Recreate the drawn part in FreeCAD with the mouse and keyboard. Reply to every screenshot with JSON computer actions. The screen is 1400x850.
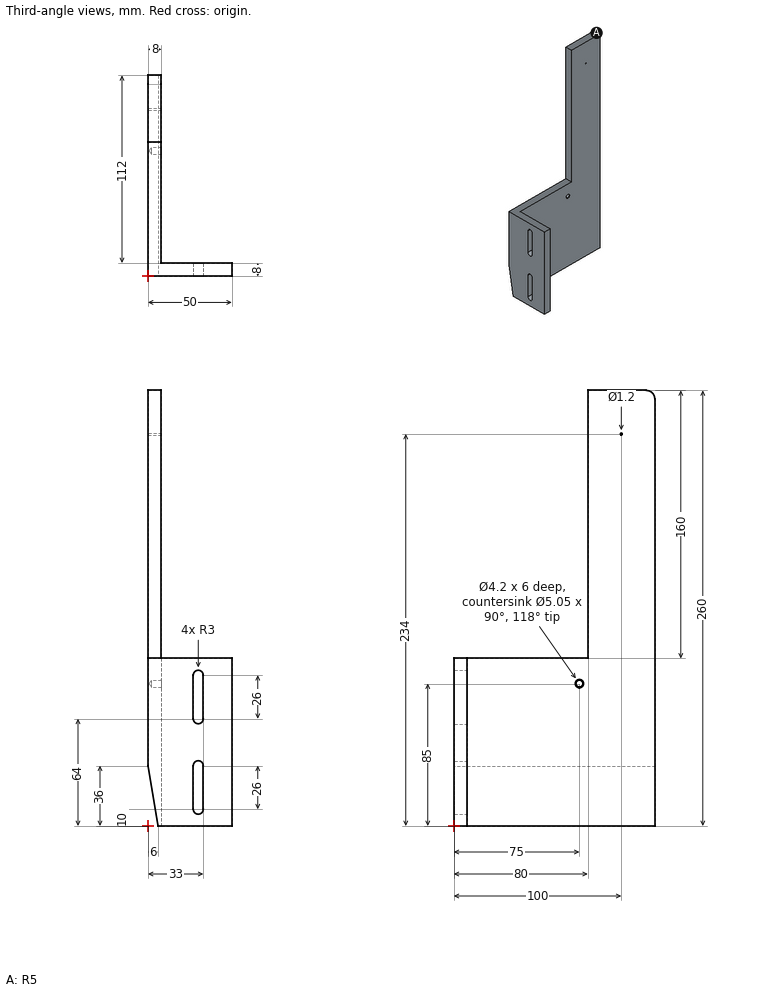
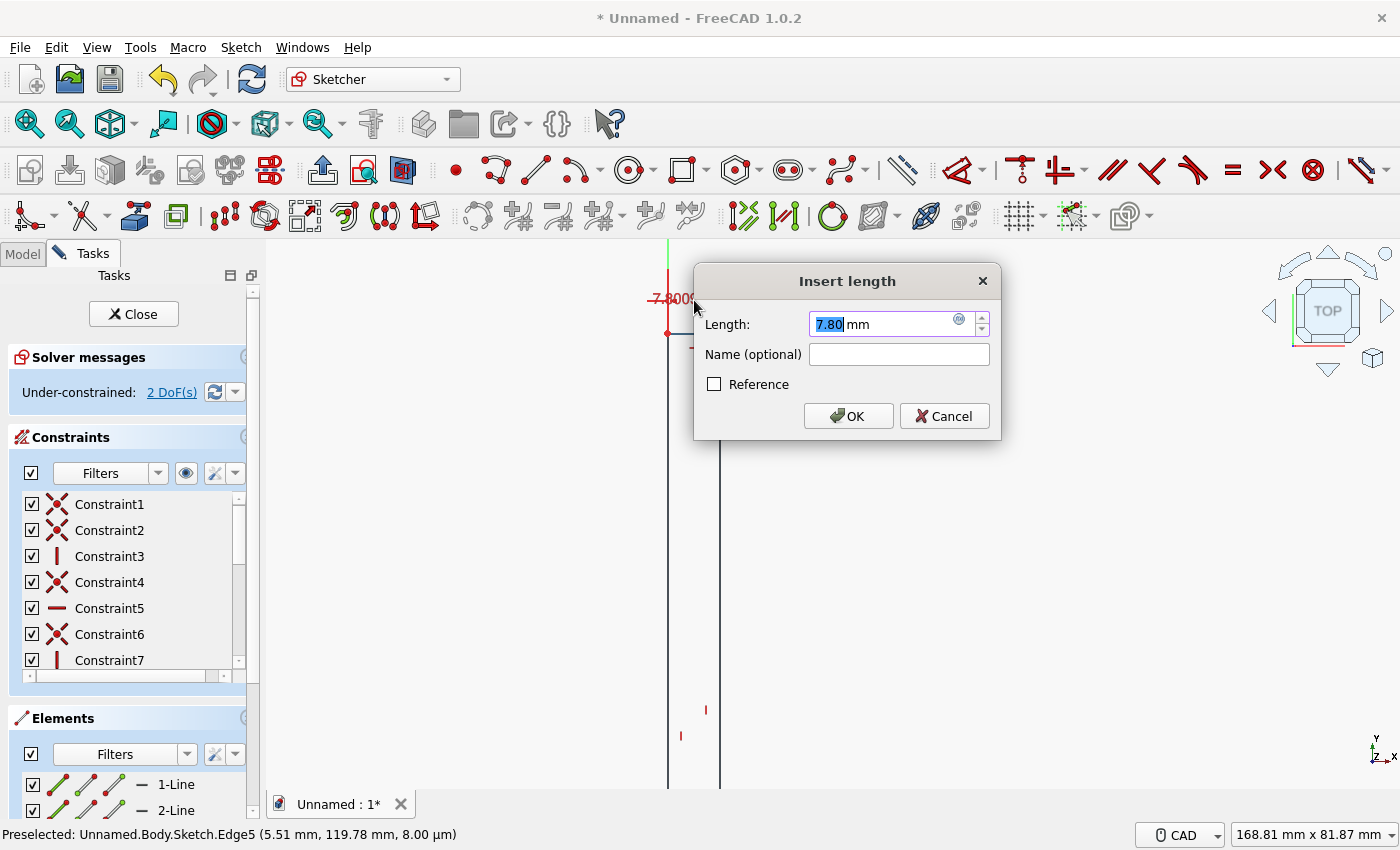
{"action": "type", "text": "8"}
{"action": "key", "text": "Return"}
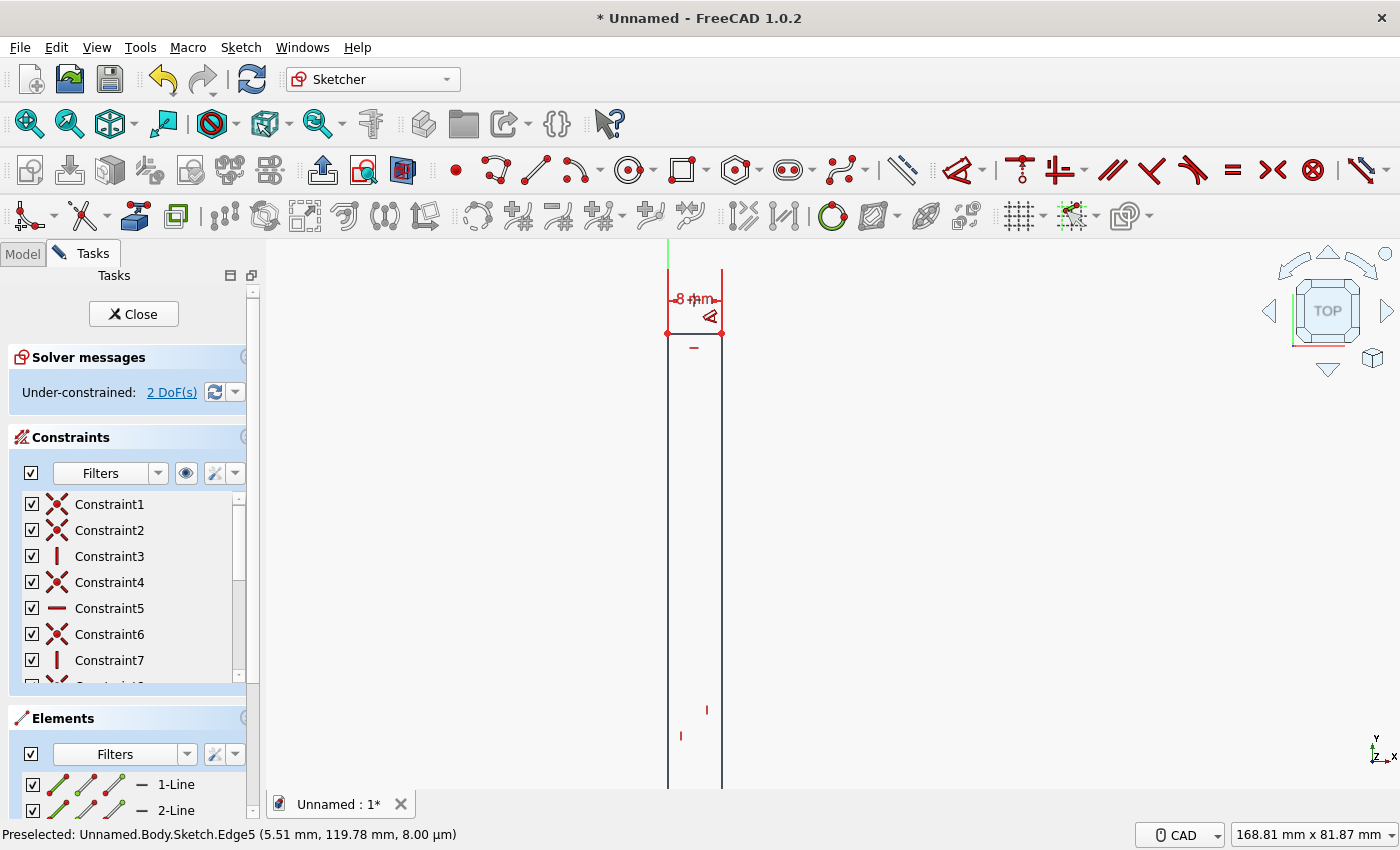
{"action": "scroll", "coordinate": [706, 333], "scroll_direction": "down", "scroll_amount": 4}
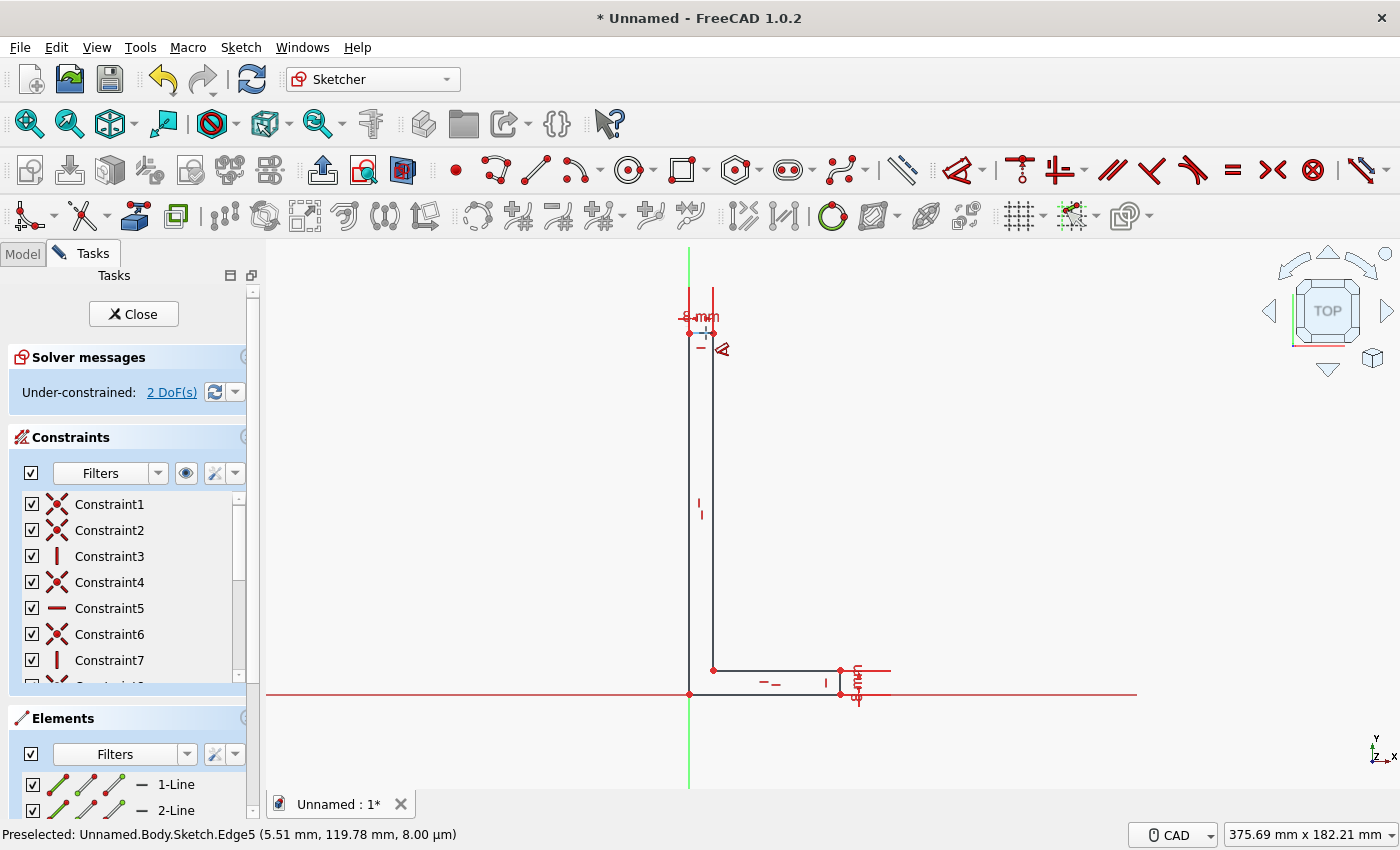
{"action": "left_click", "coordinate": [735, 695]}
{"action": "left_click", "coordinate": [765, 729]}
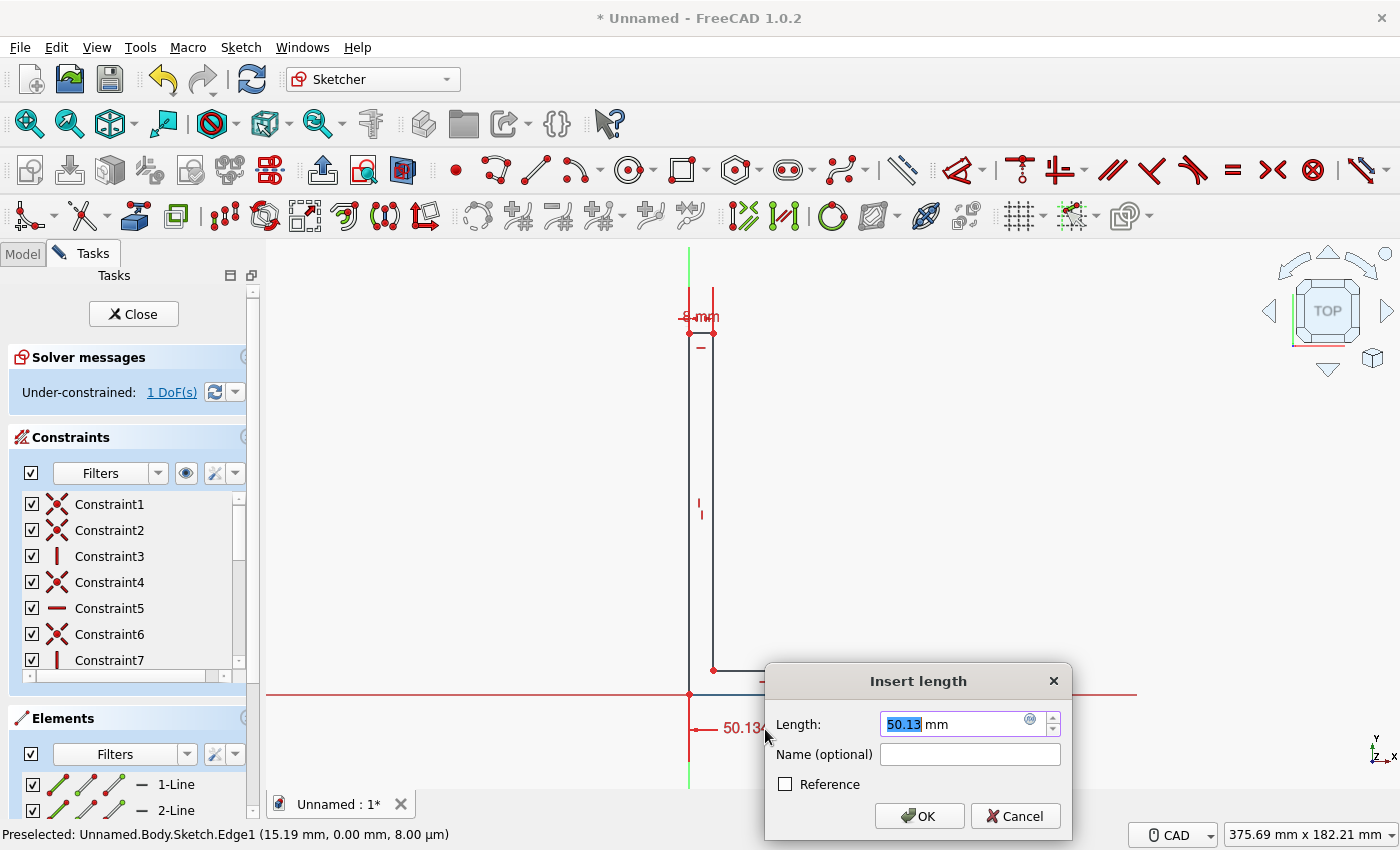
{"action": "type", "text": "50"}
{"action": "key", "text": "Return"}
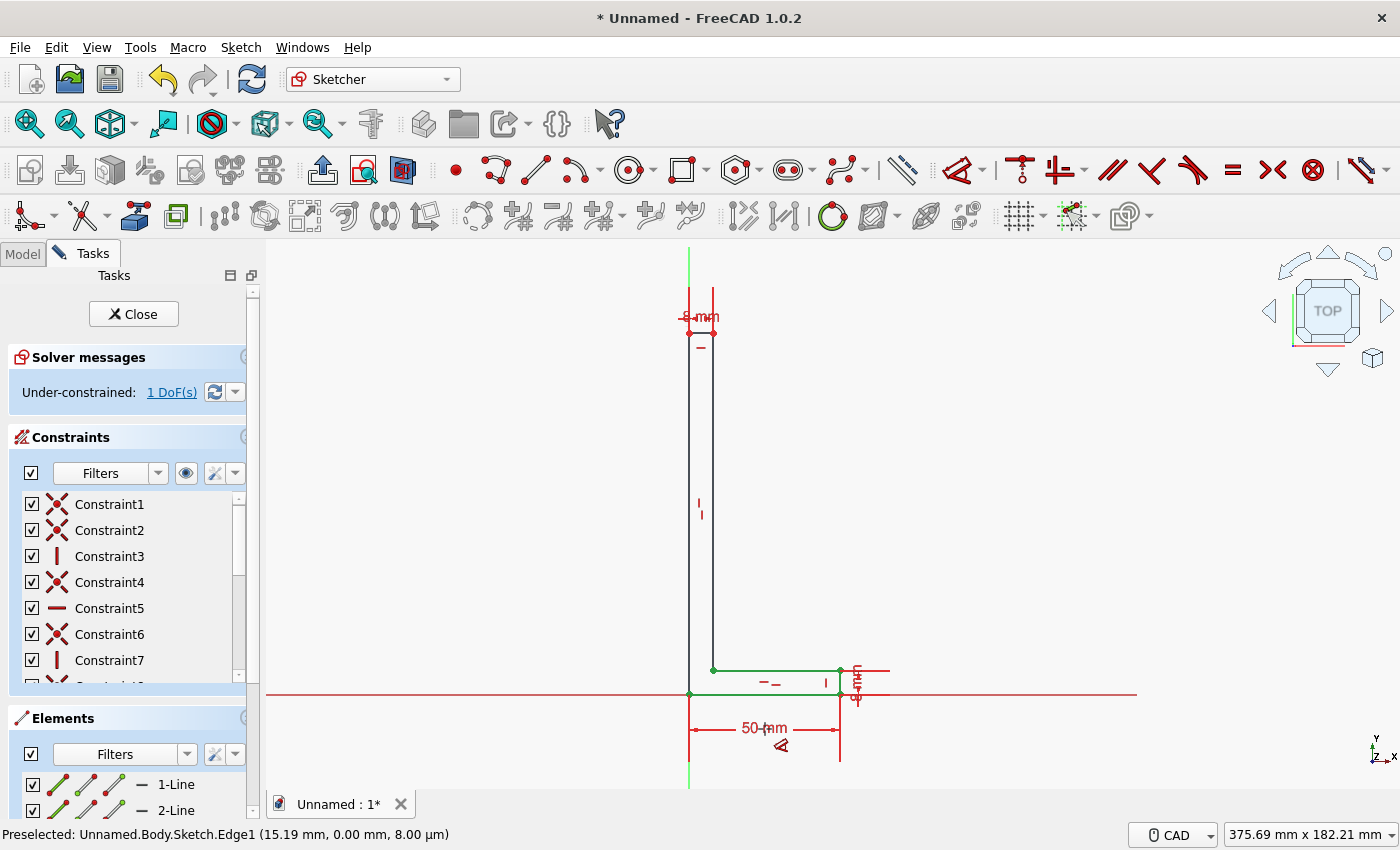
{"action": "left_click", "coordinate": [713, 570]}
{"action": "left_click", "coordinate": [747, 502]}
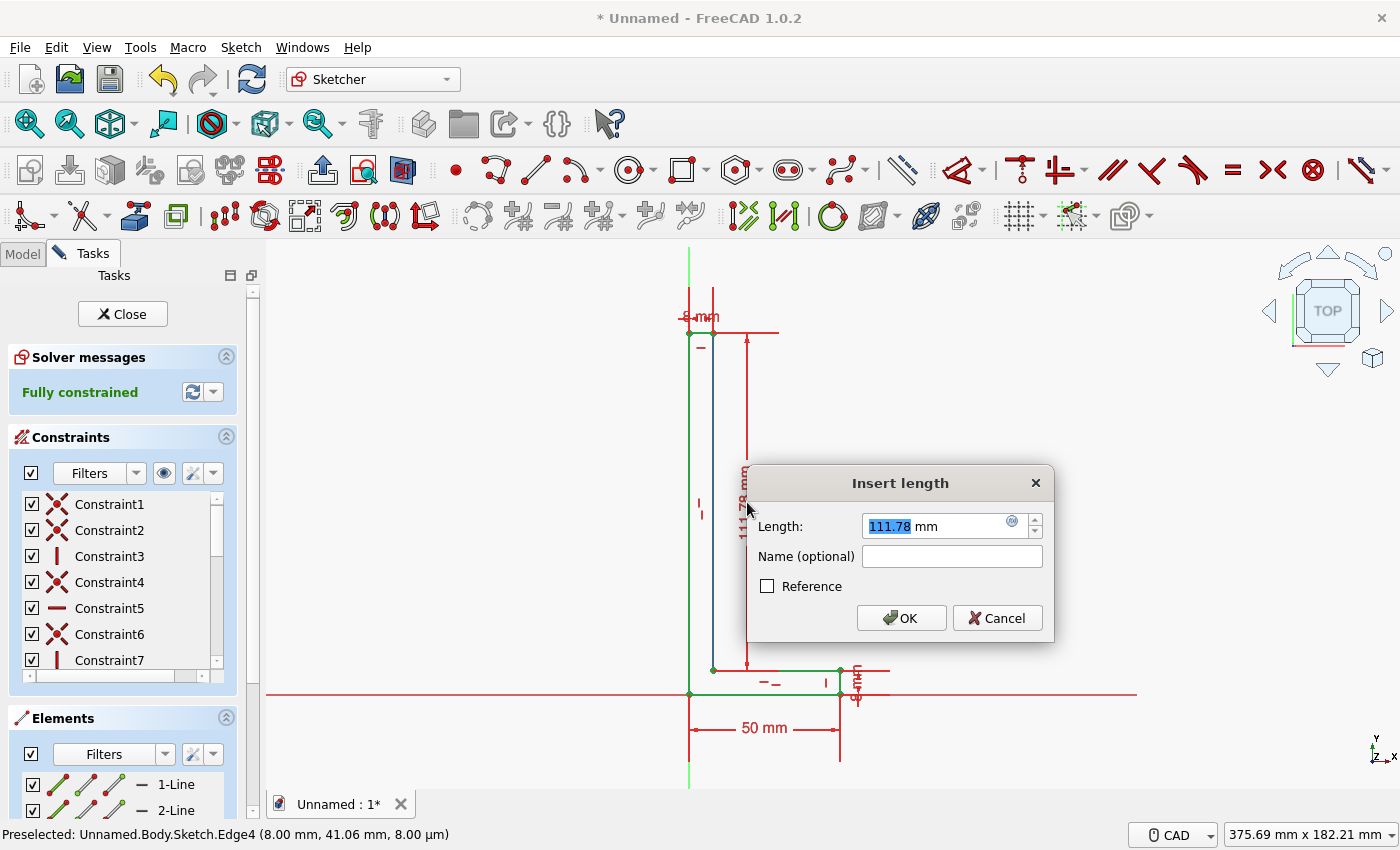
{"action": "type", "text": "112"}
{"action": "key", "text": "Return"}
{"action": "key", "text": "Escape"}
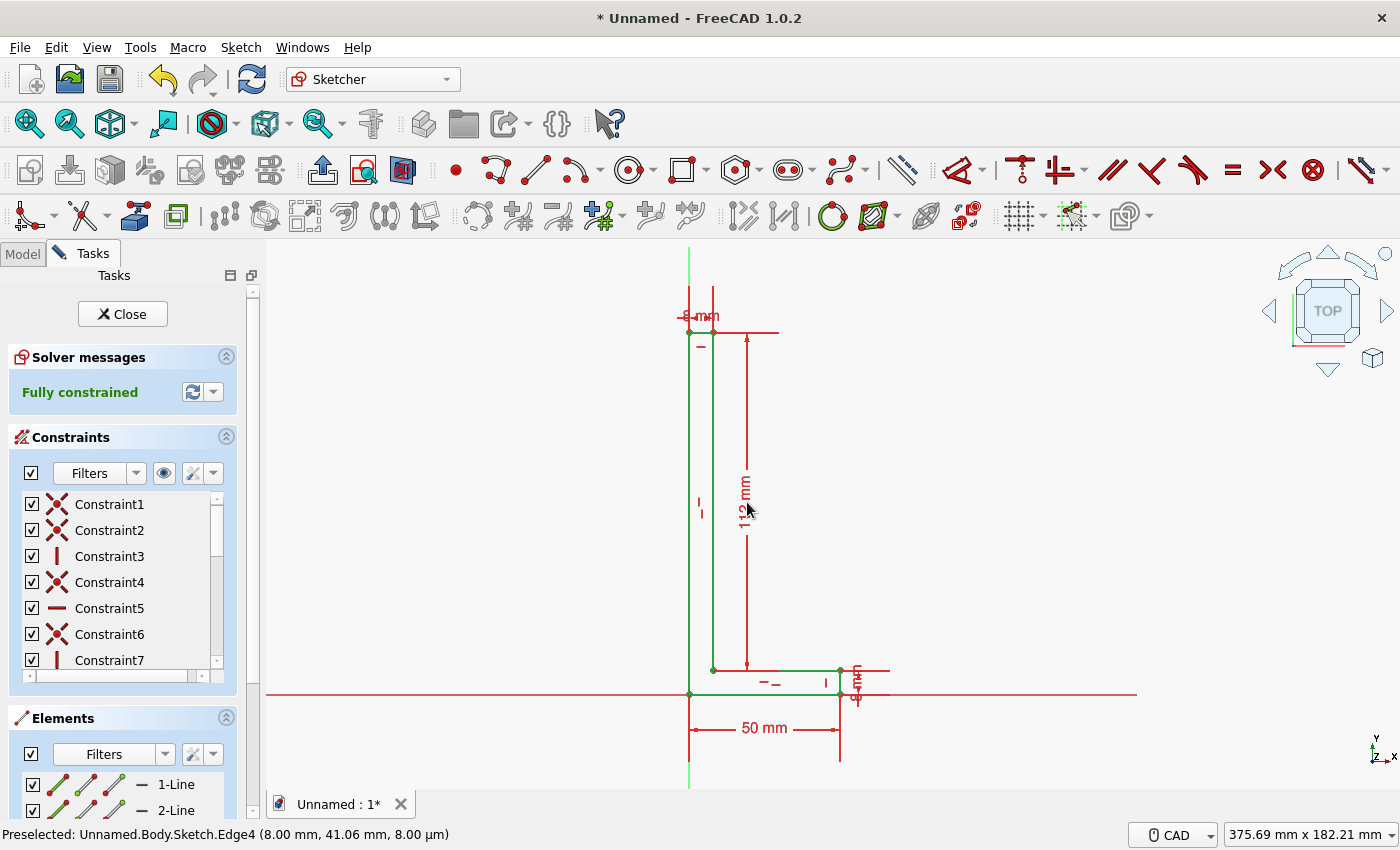
{"action": "left_click", "coordinate": [123, 314]}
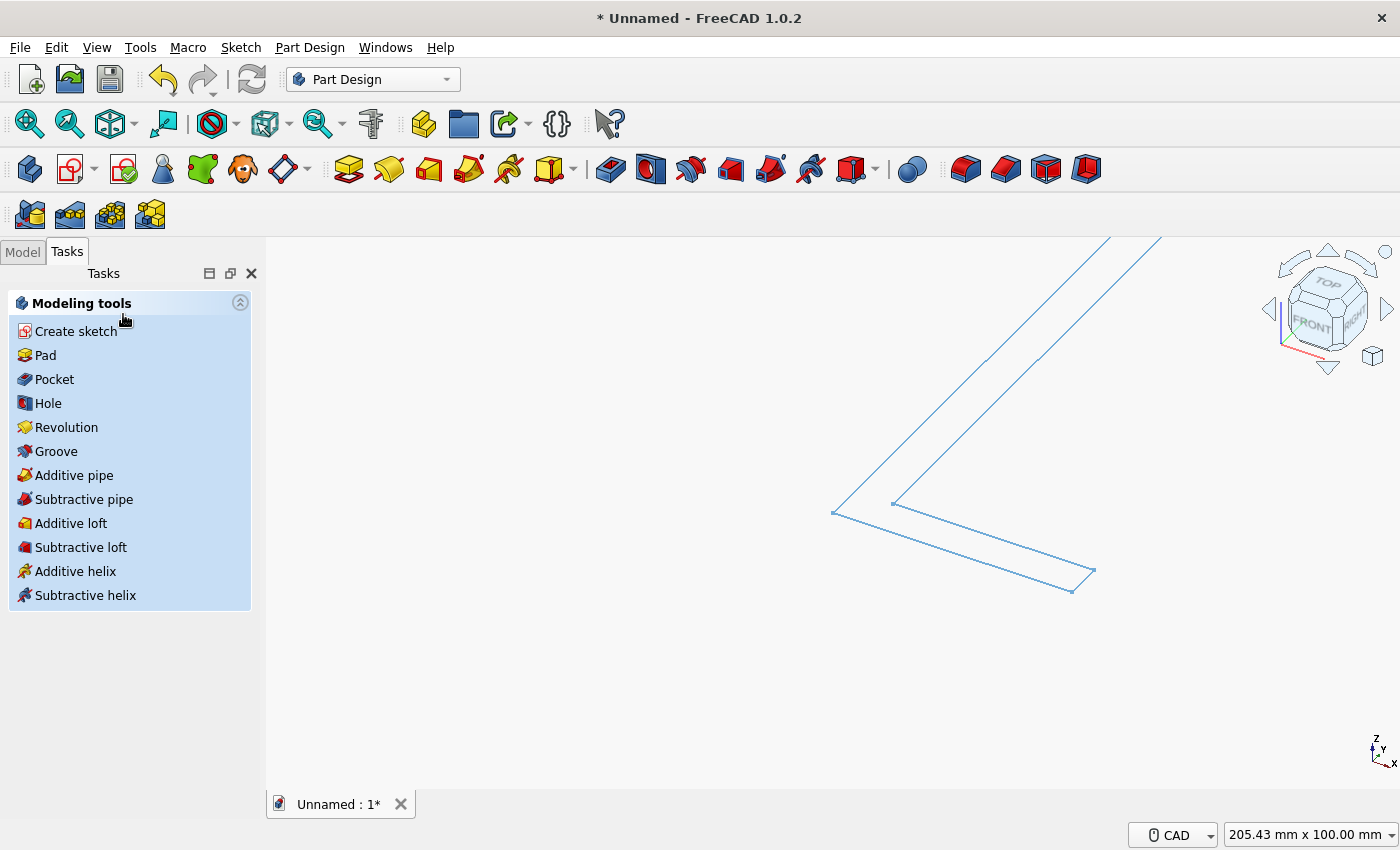
{"action": "left_click", "coordinate": [350, 170]}